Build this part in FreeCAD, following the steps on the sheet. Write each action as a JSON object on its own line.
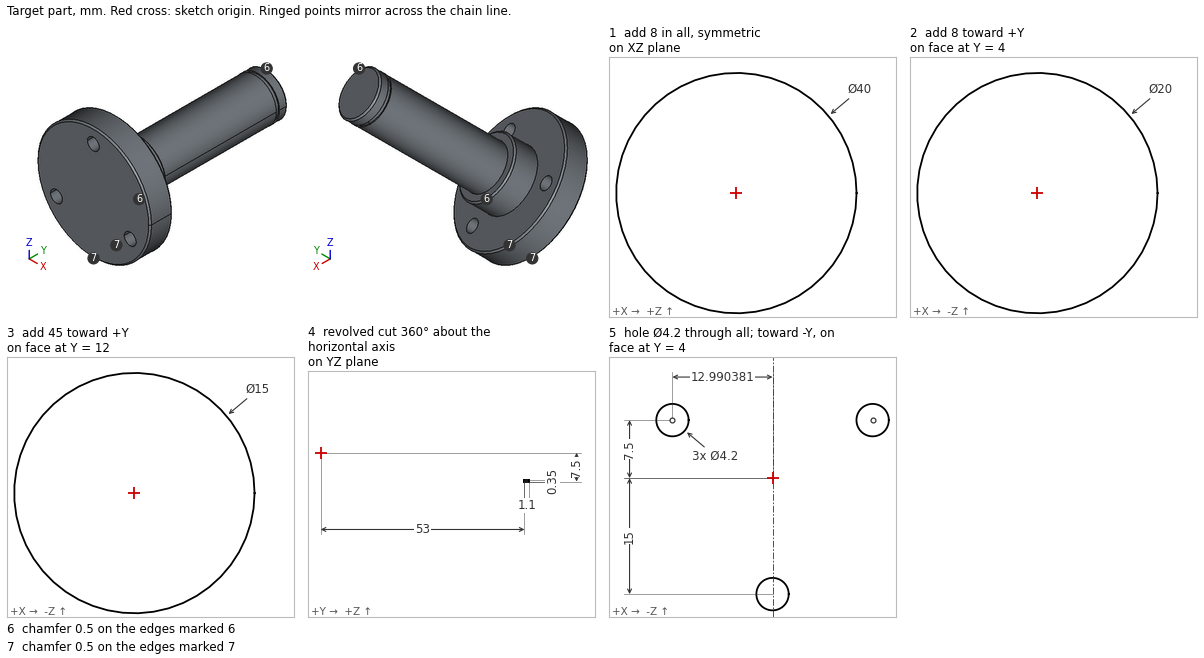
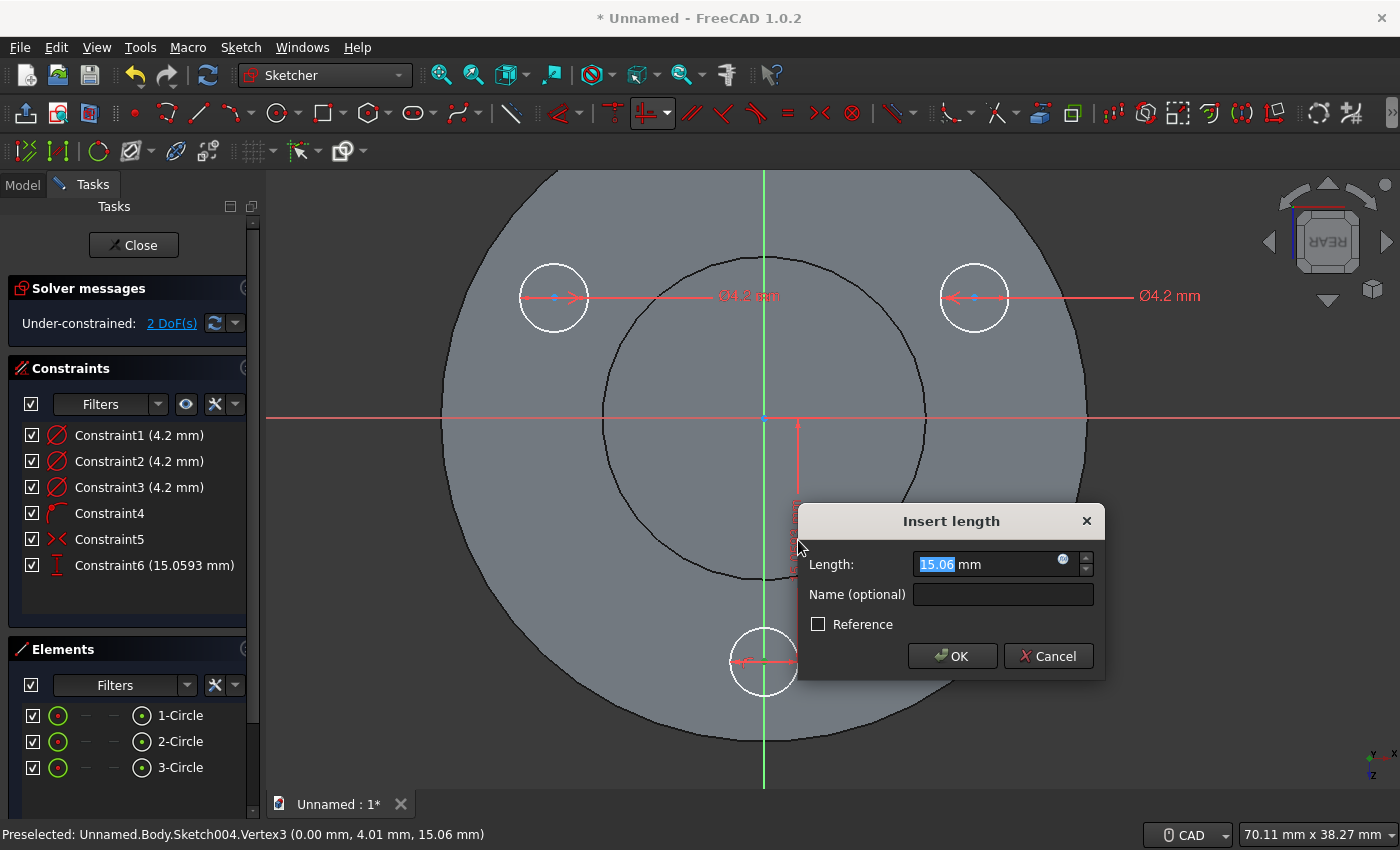
{"action": "type", "text": "15"}
{"action": "key", "text": "Return"}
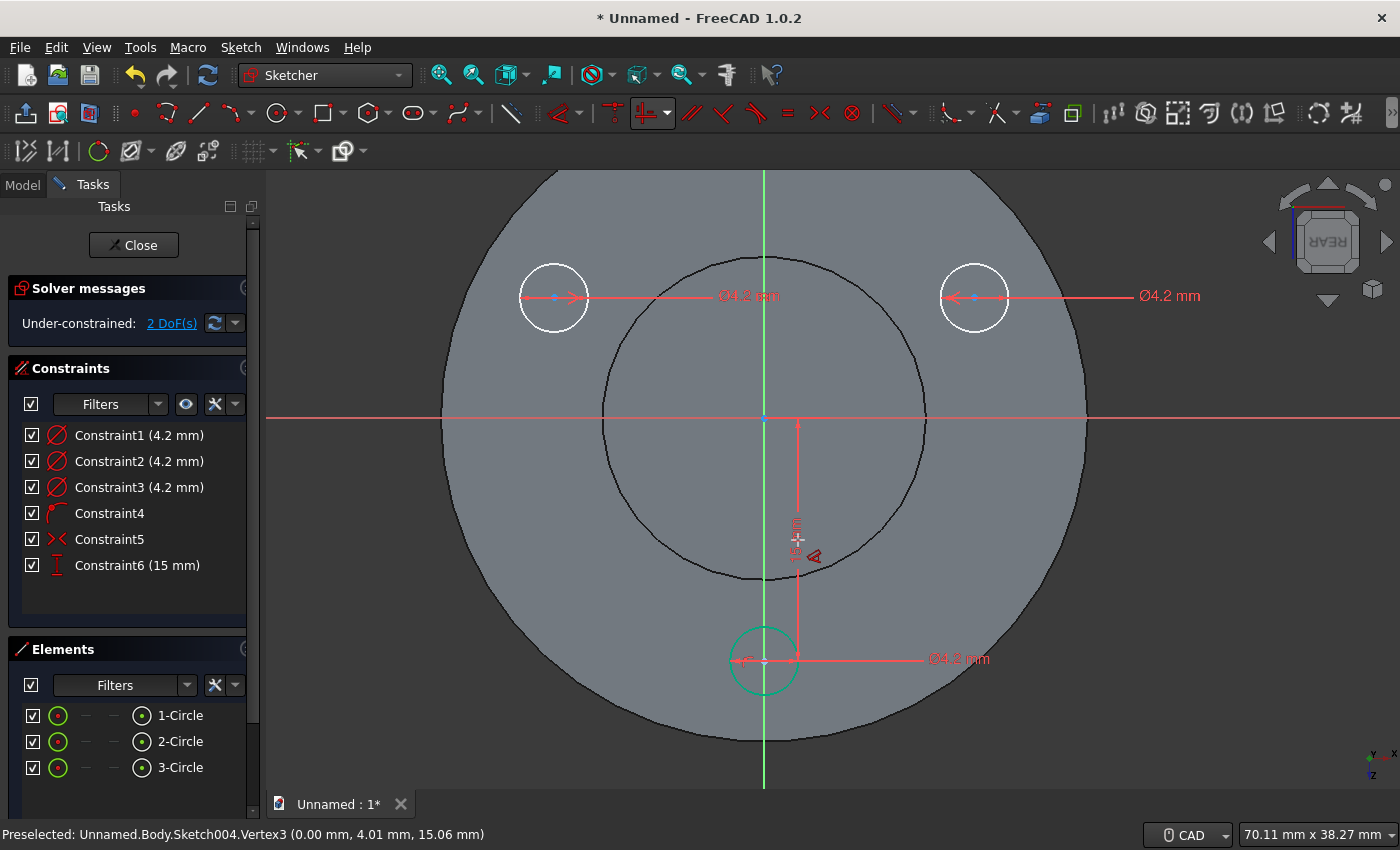
{"action": "left_click", "coordinate": [554, 298]}
{"action": "left_click", "coordinate": [520, 358]}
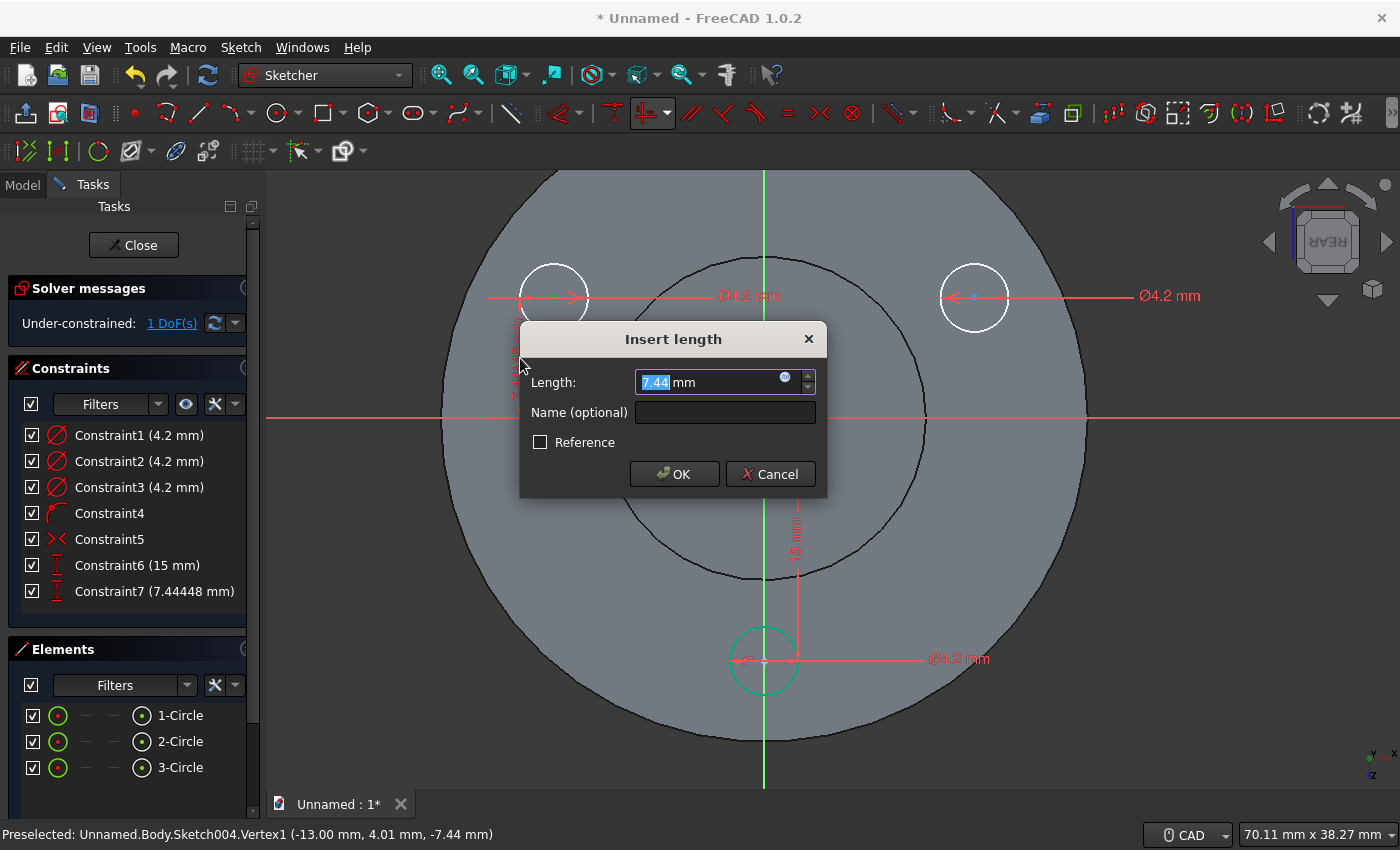
{"action": "type", "text": "7.5"}
{"action": "key", "text": "Return"}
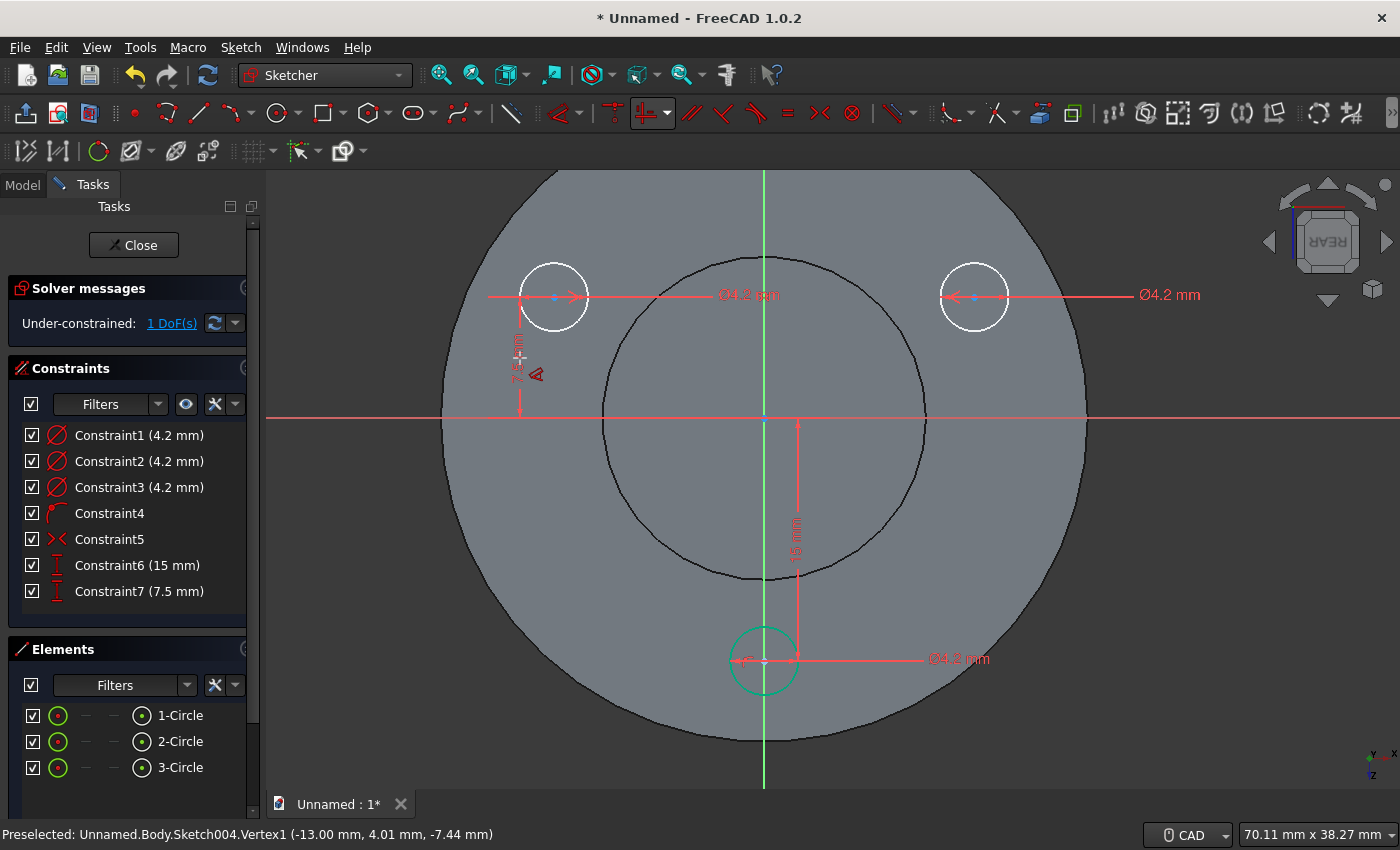
{"action": "left_click", "coordinate": [554, 297]}
{"action": "left_click", "coordinate": [659, 263]}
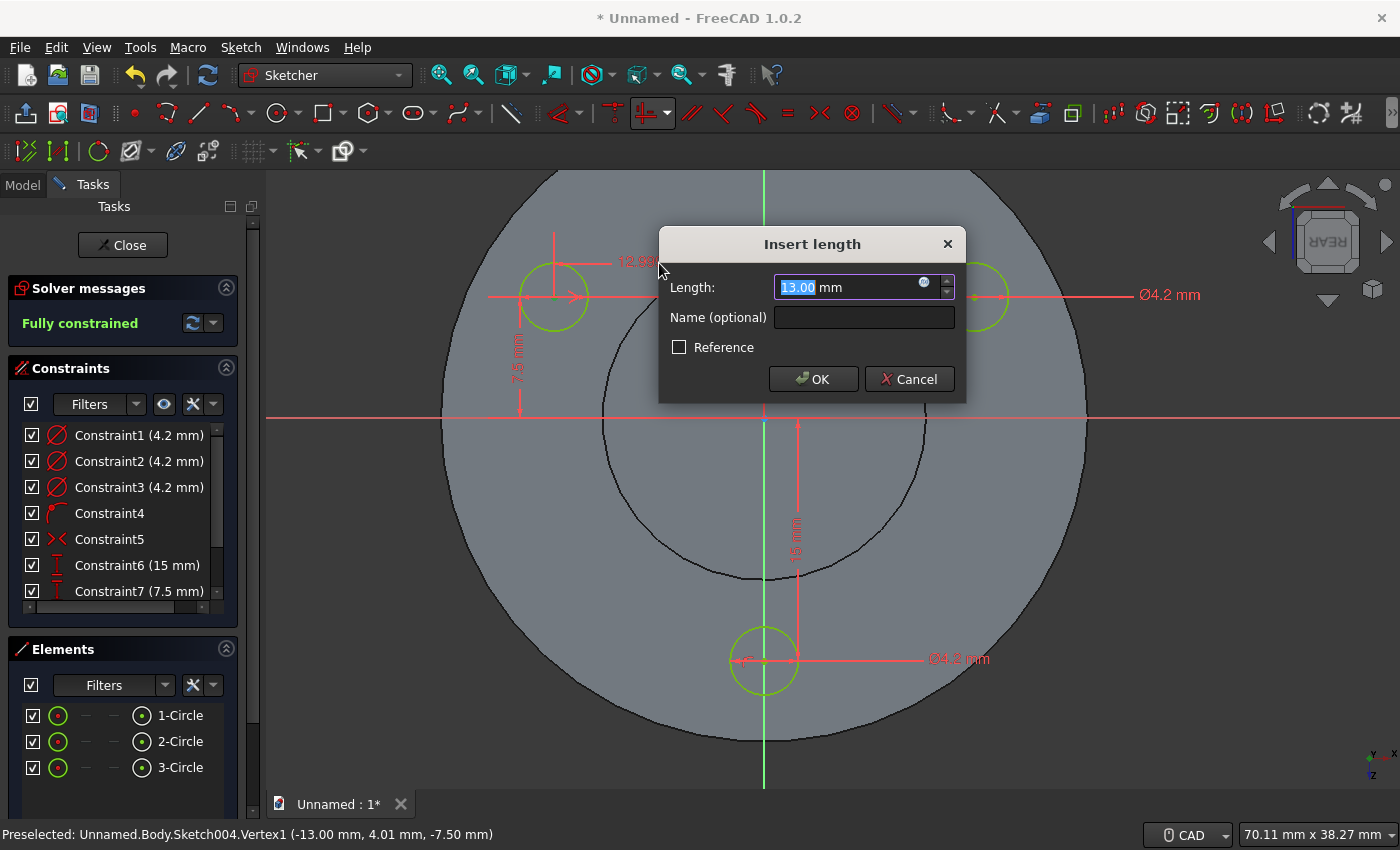
{"action": "type", "text": "12.990381"}
{"action": "key", "text": "Return"}
{"action": "key", "text": "Escape"}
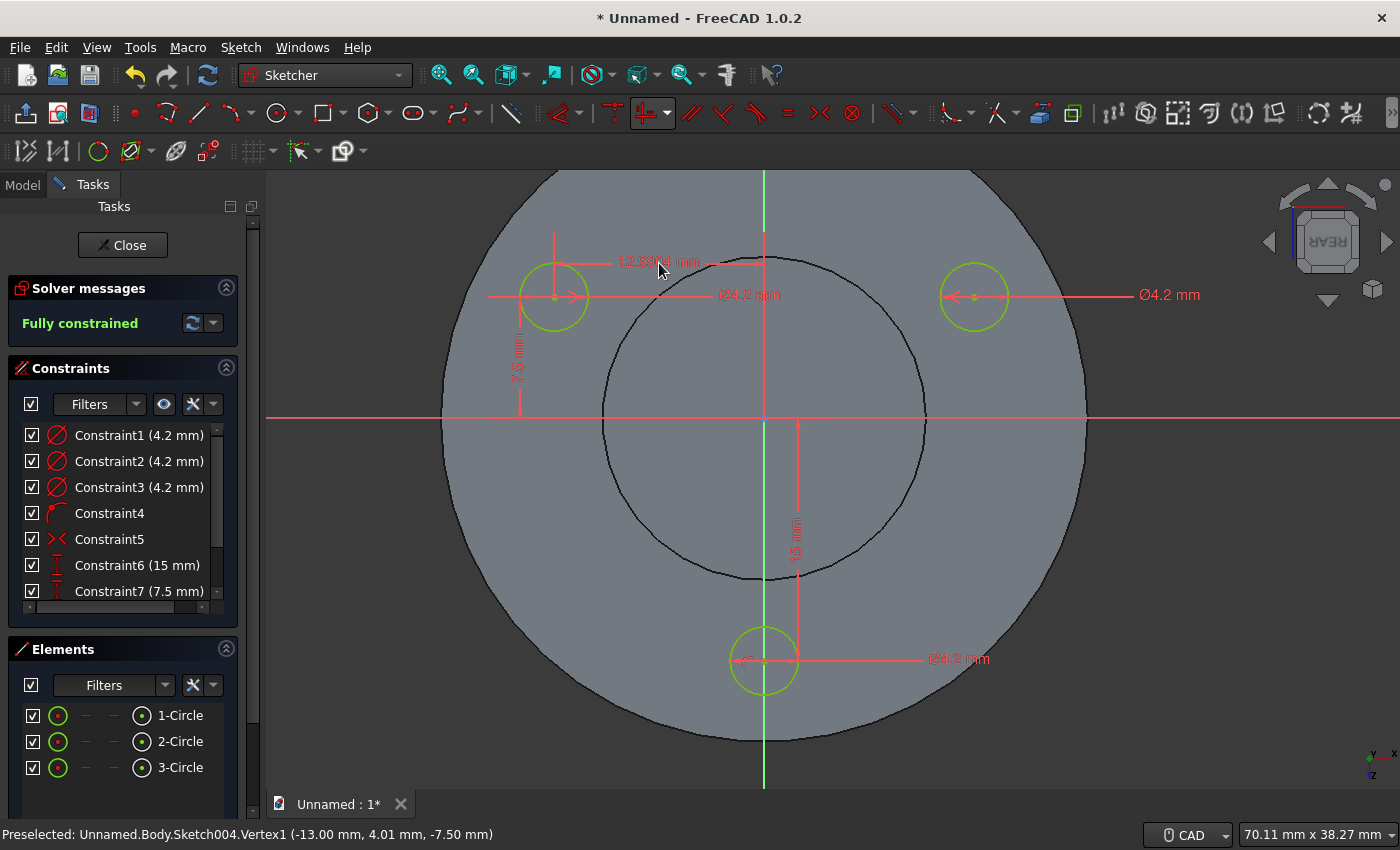
{"action": "left_click", "coordinate": [123, 245]}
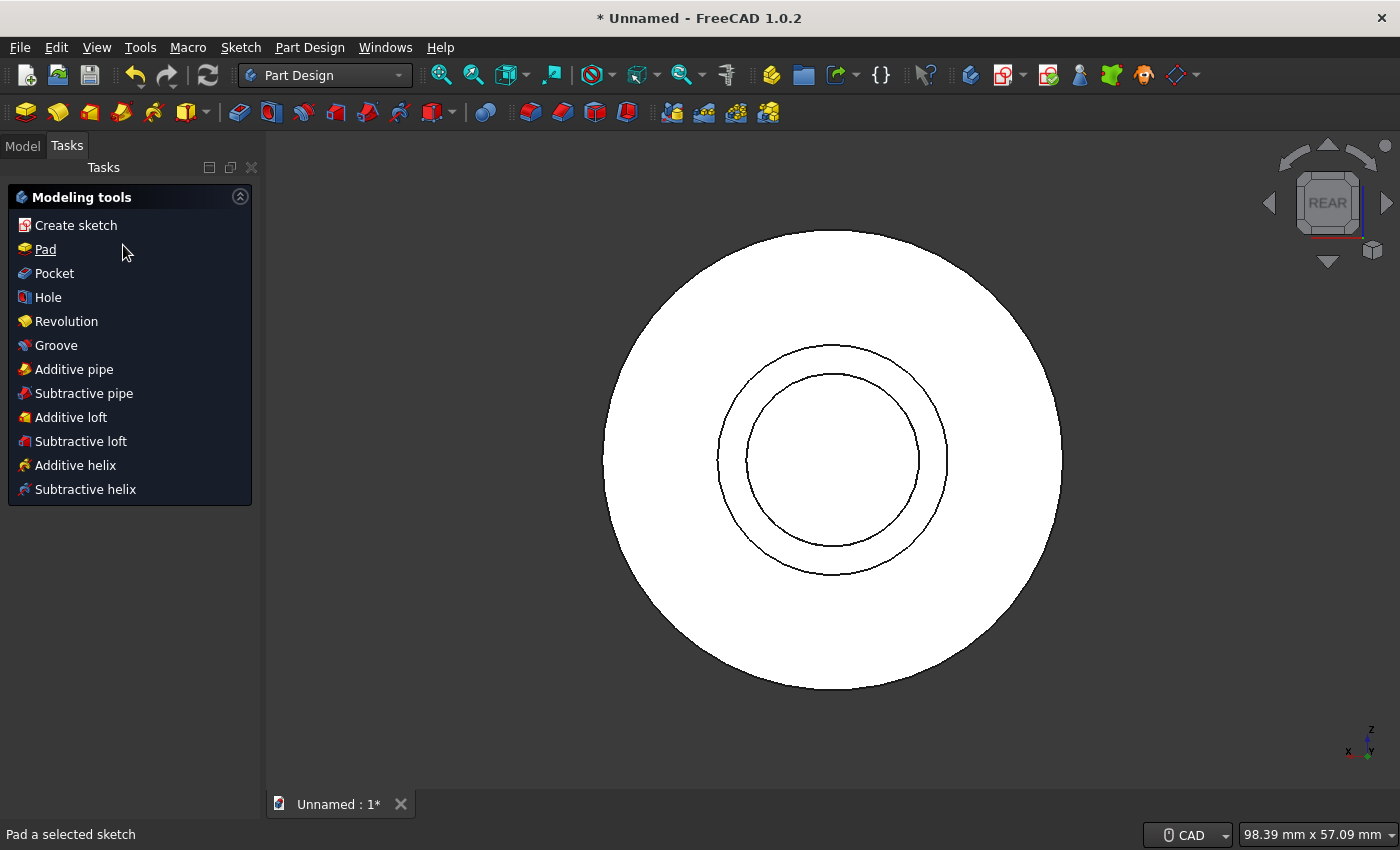
{"action": "left_click", "coordinate": [272, 112]}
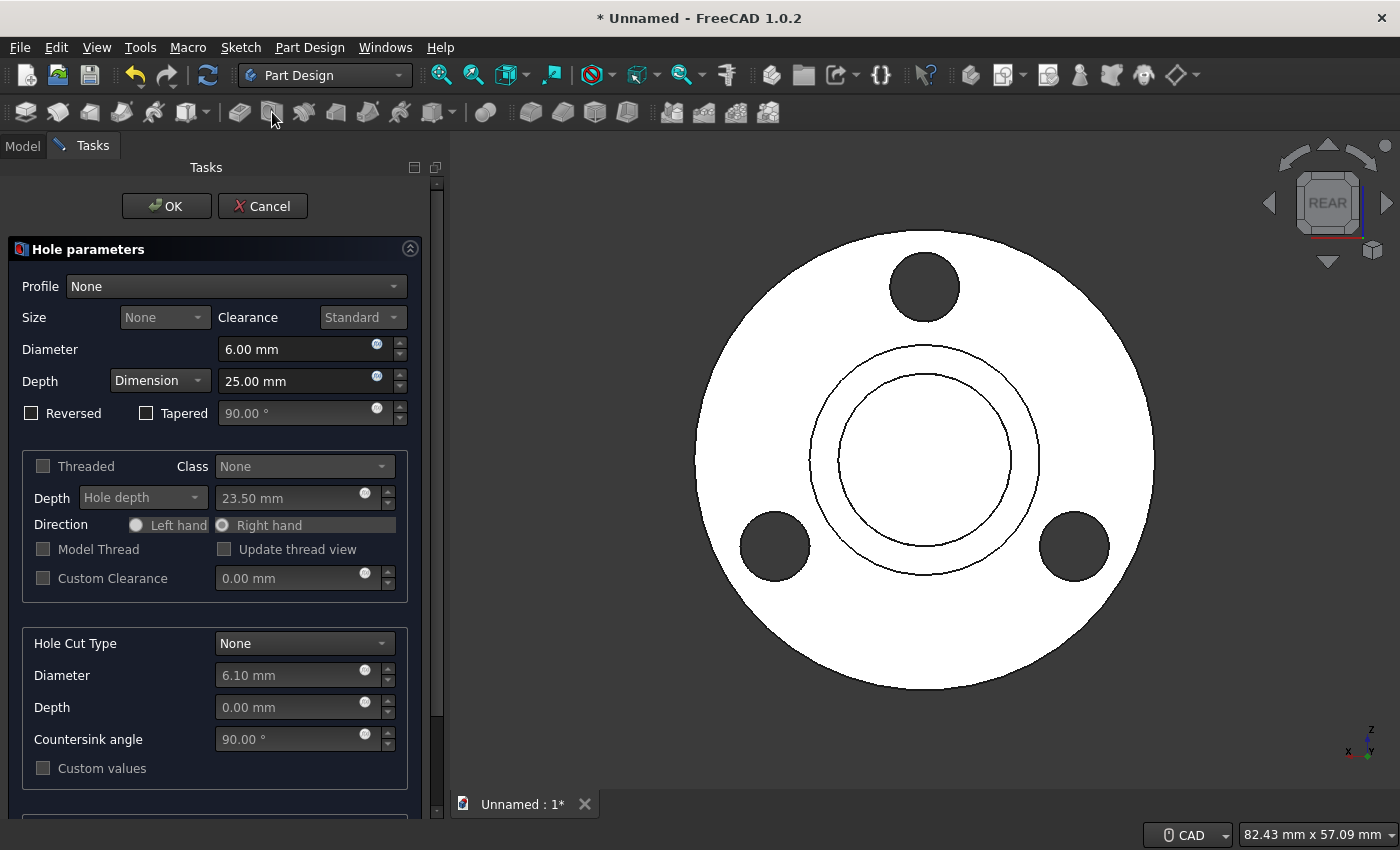
{"action": "triple_click", "coordinate": [305, 349]}